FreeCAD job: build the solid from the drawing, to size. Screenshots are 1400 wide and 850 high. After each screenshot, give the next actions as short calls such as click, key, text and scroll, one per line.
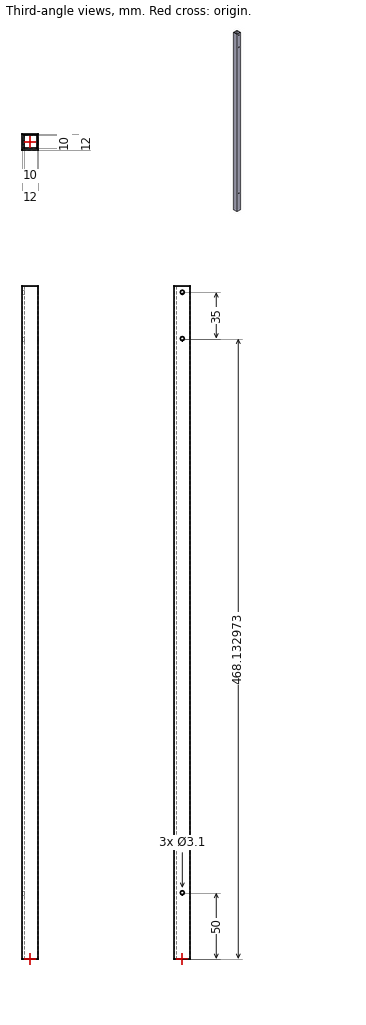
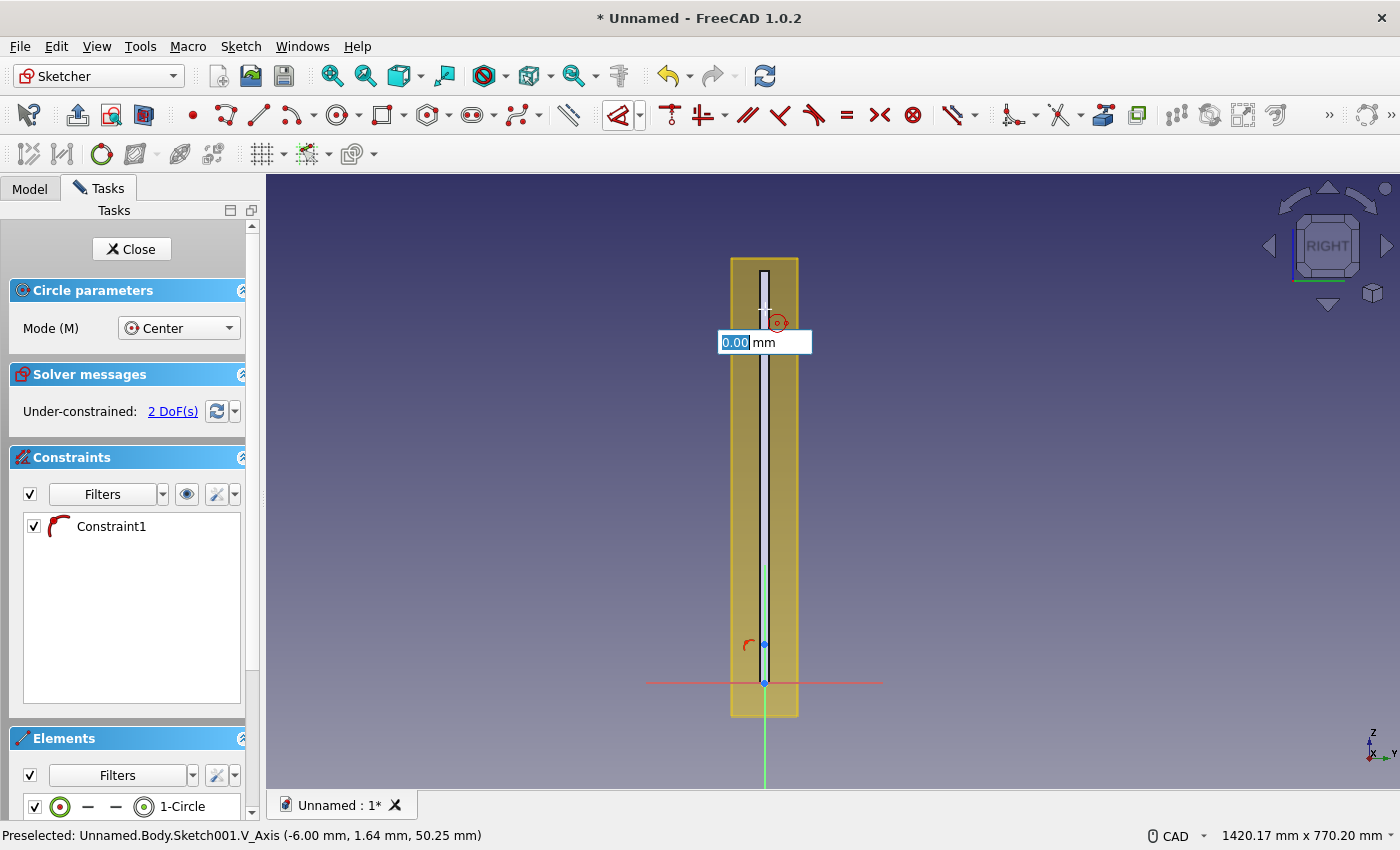
scroll(766, 309, up, 14)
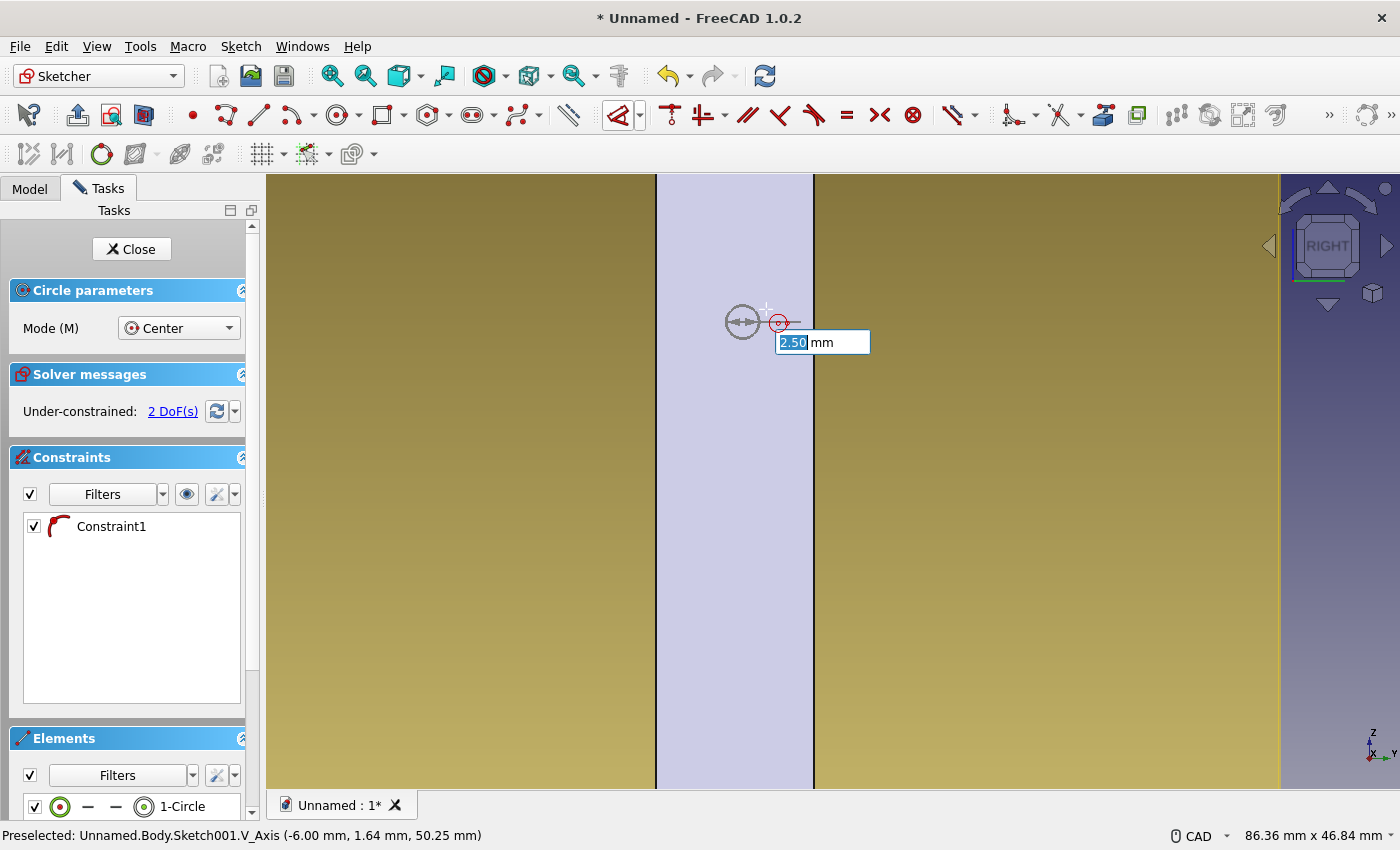
click(754, 306)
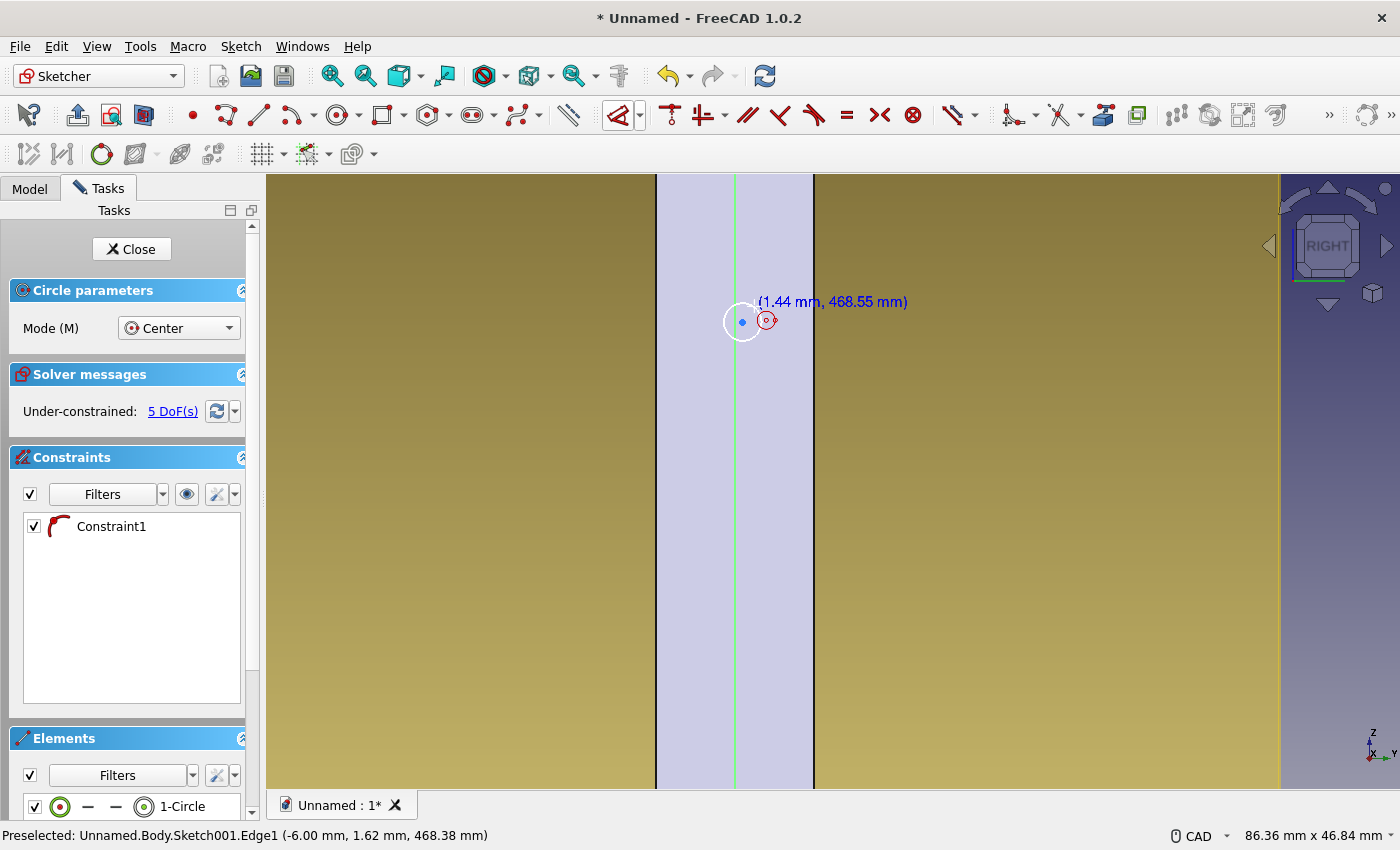
scroll(766, 309, down, 14)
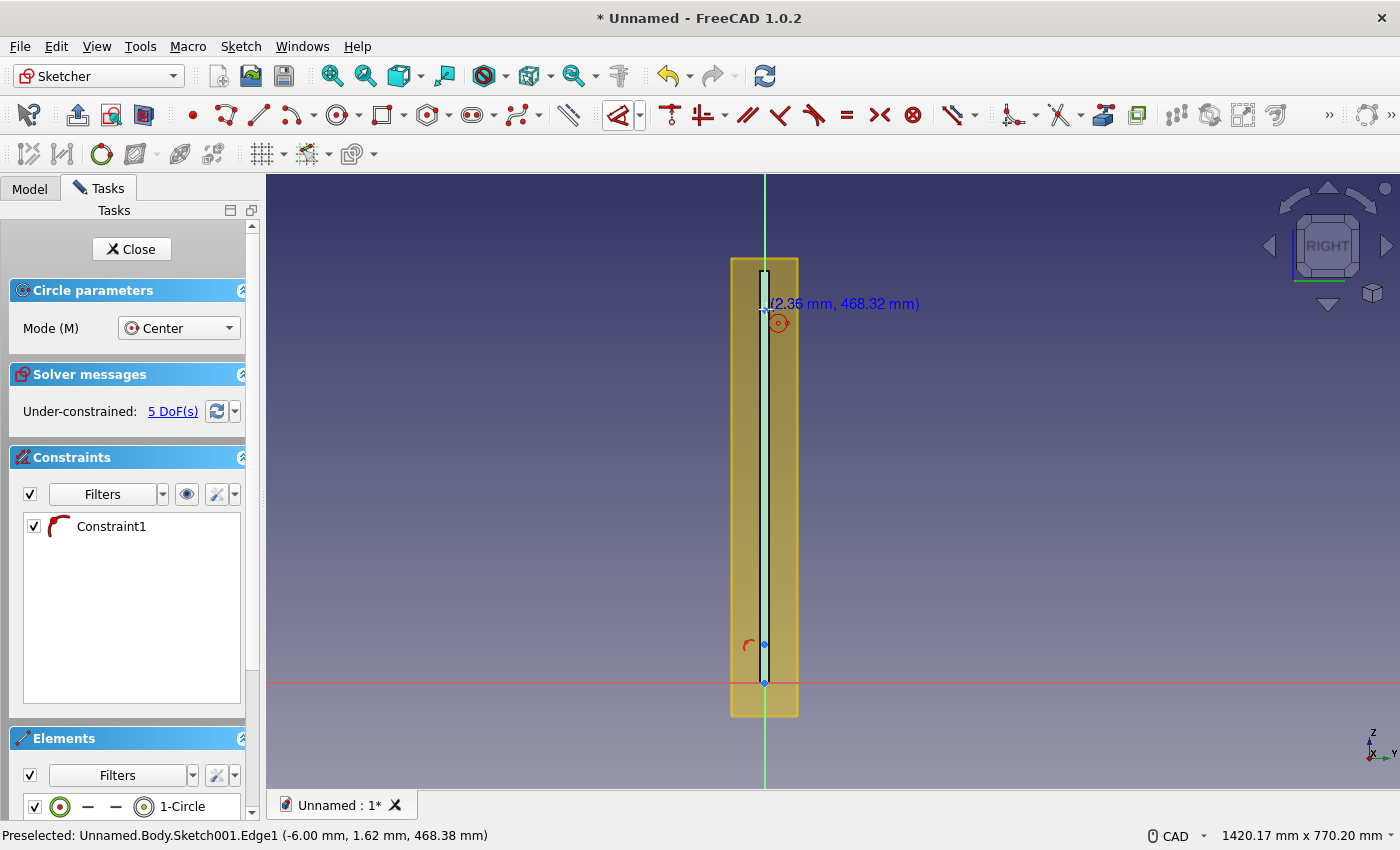
scroll(765, 281, up, 15)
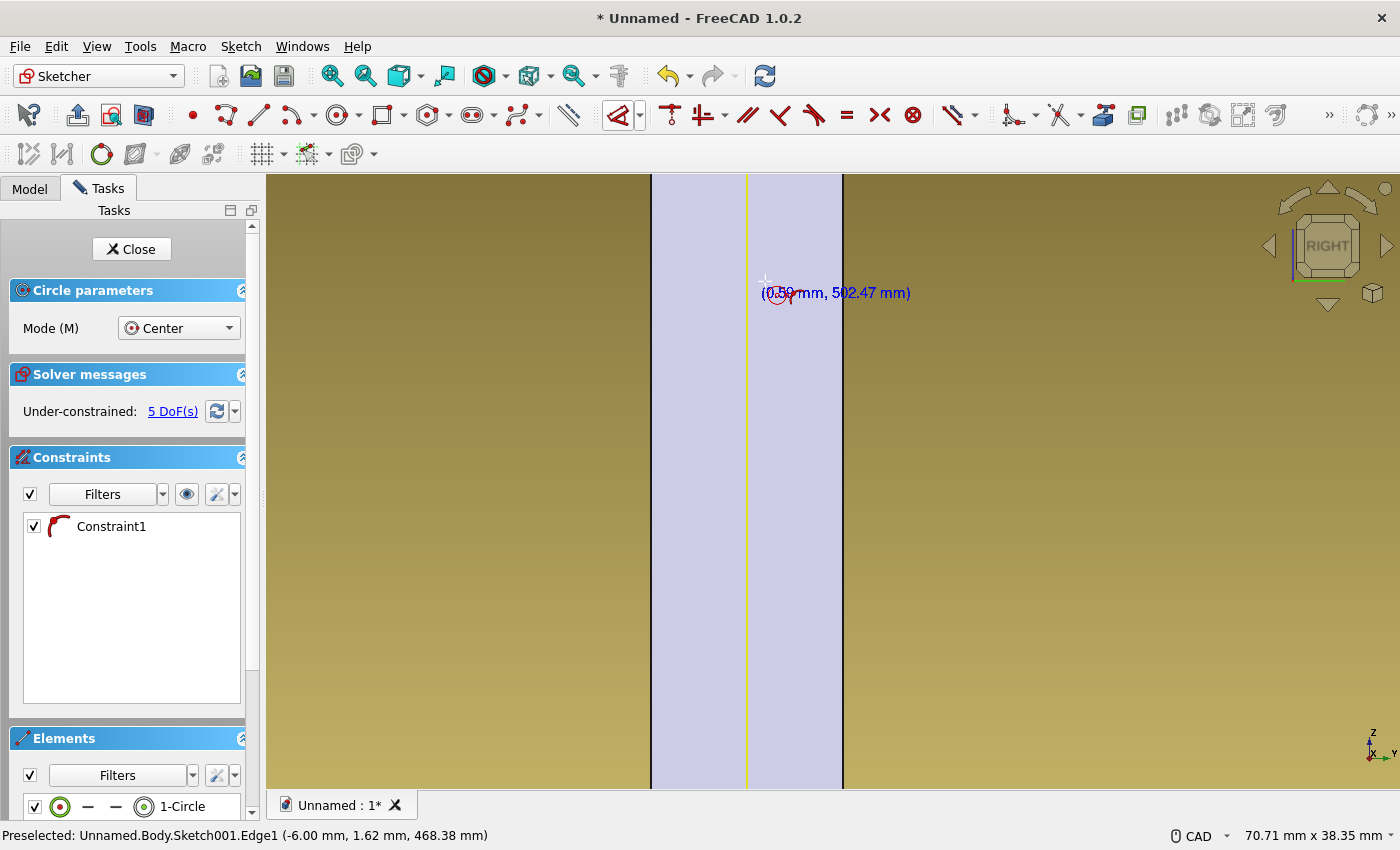
scroll(765, 281, down, 15)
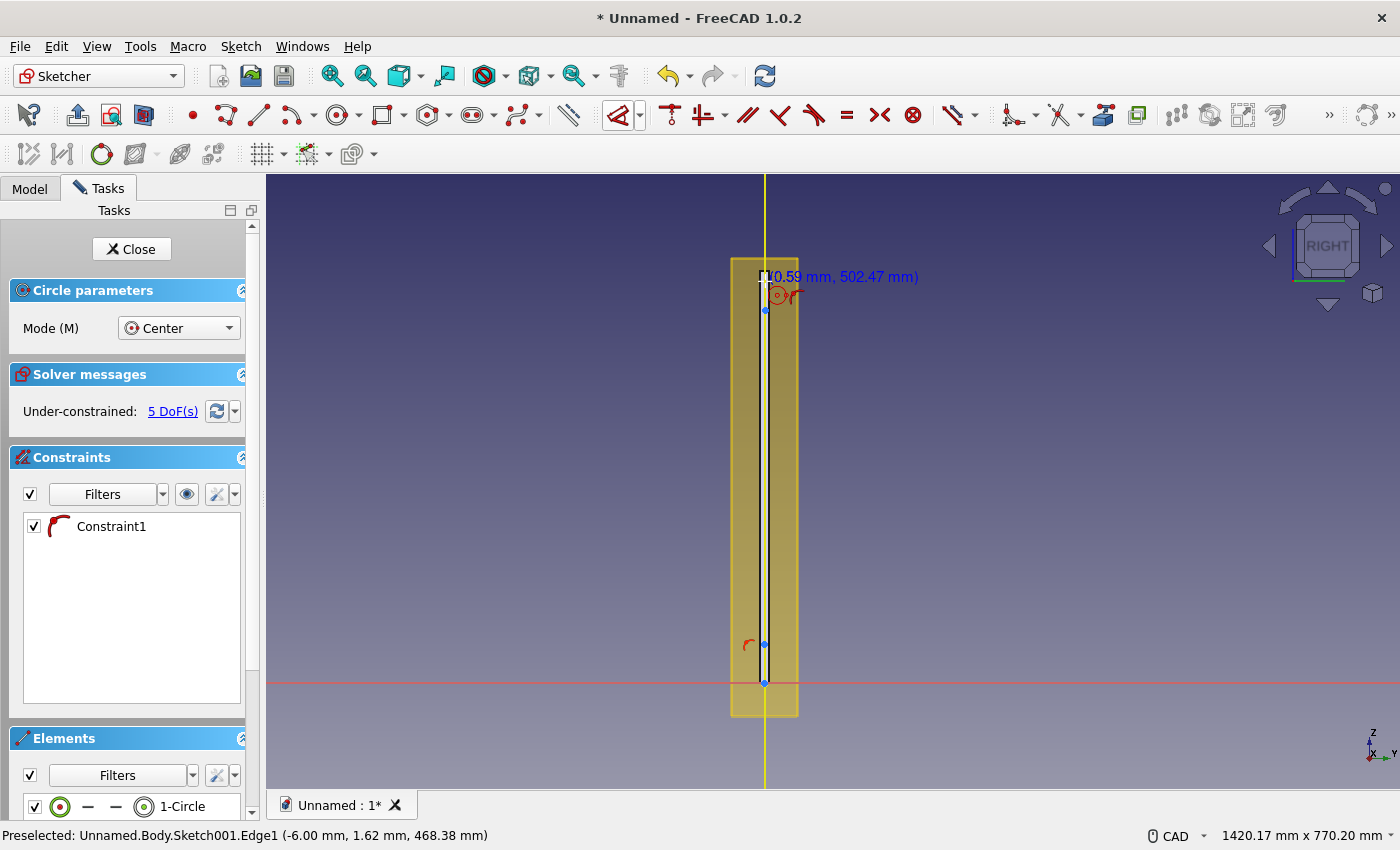
click(765, 281)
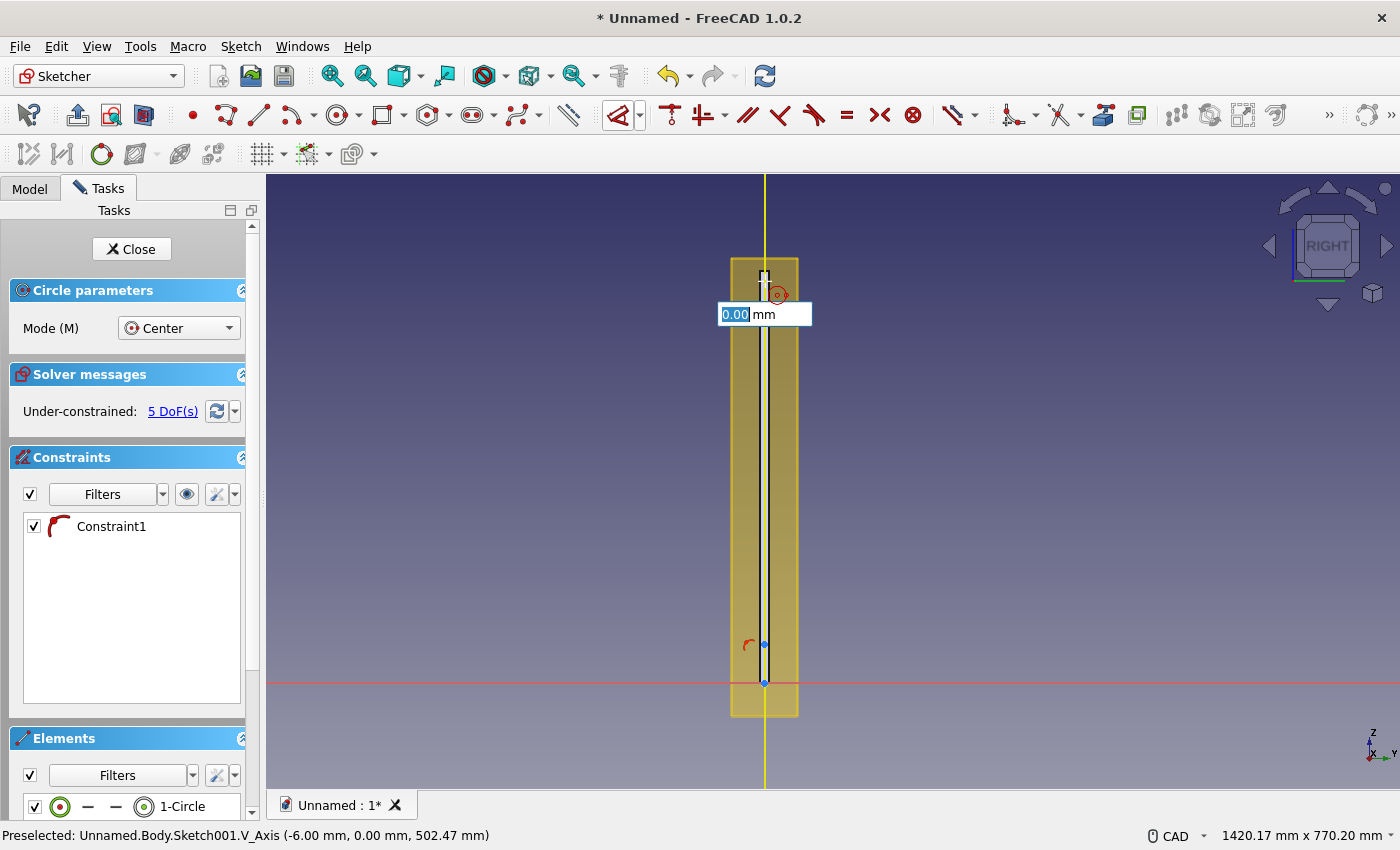
scroll(766, 281, up, 14)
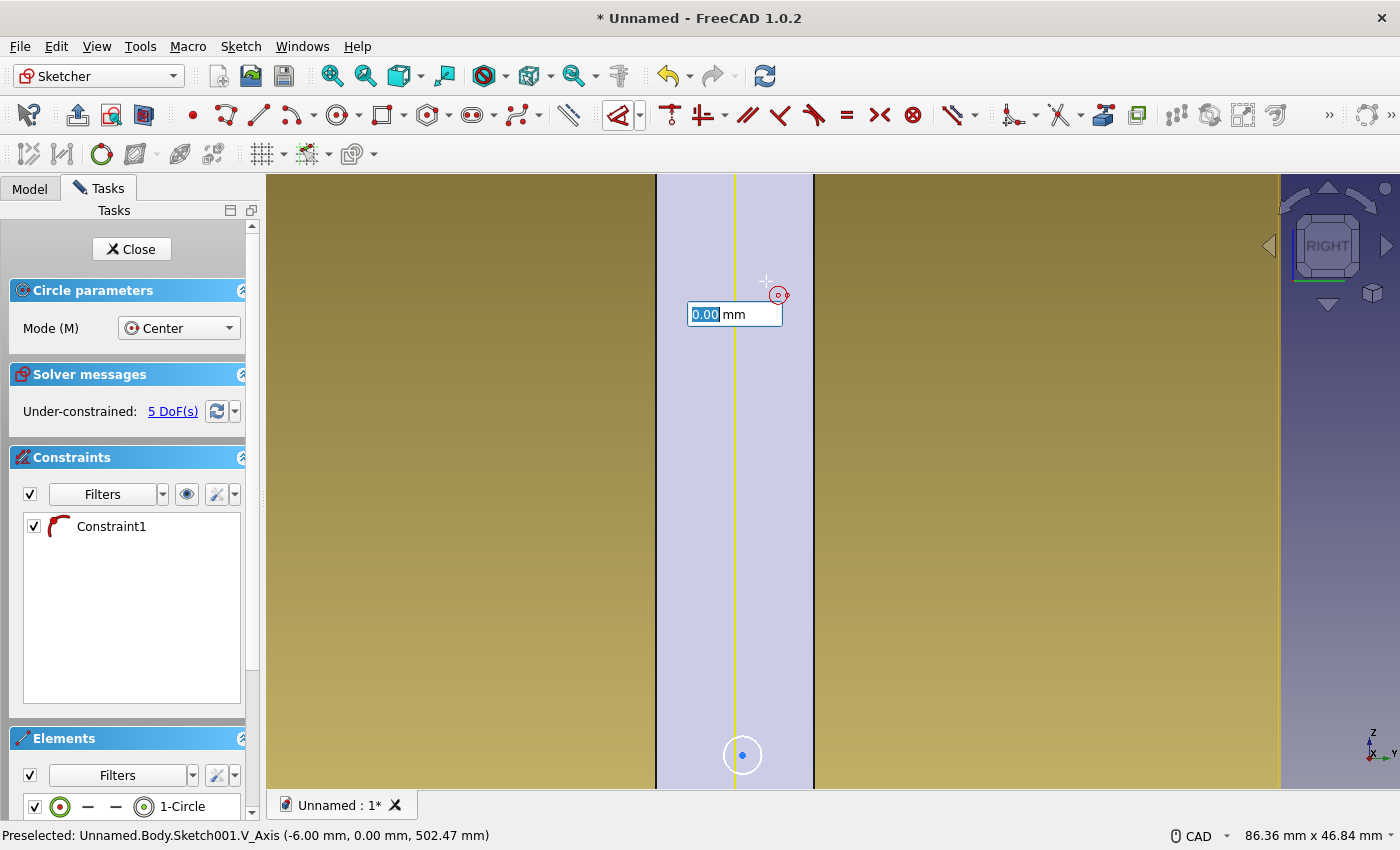
click(754, 279)
key(Escape)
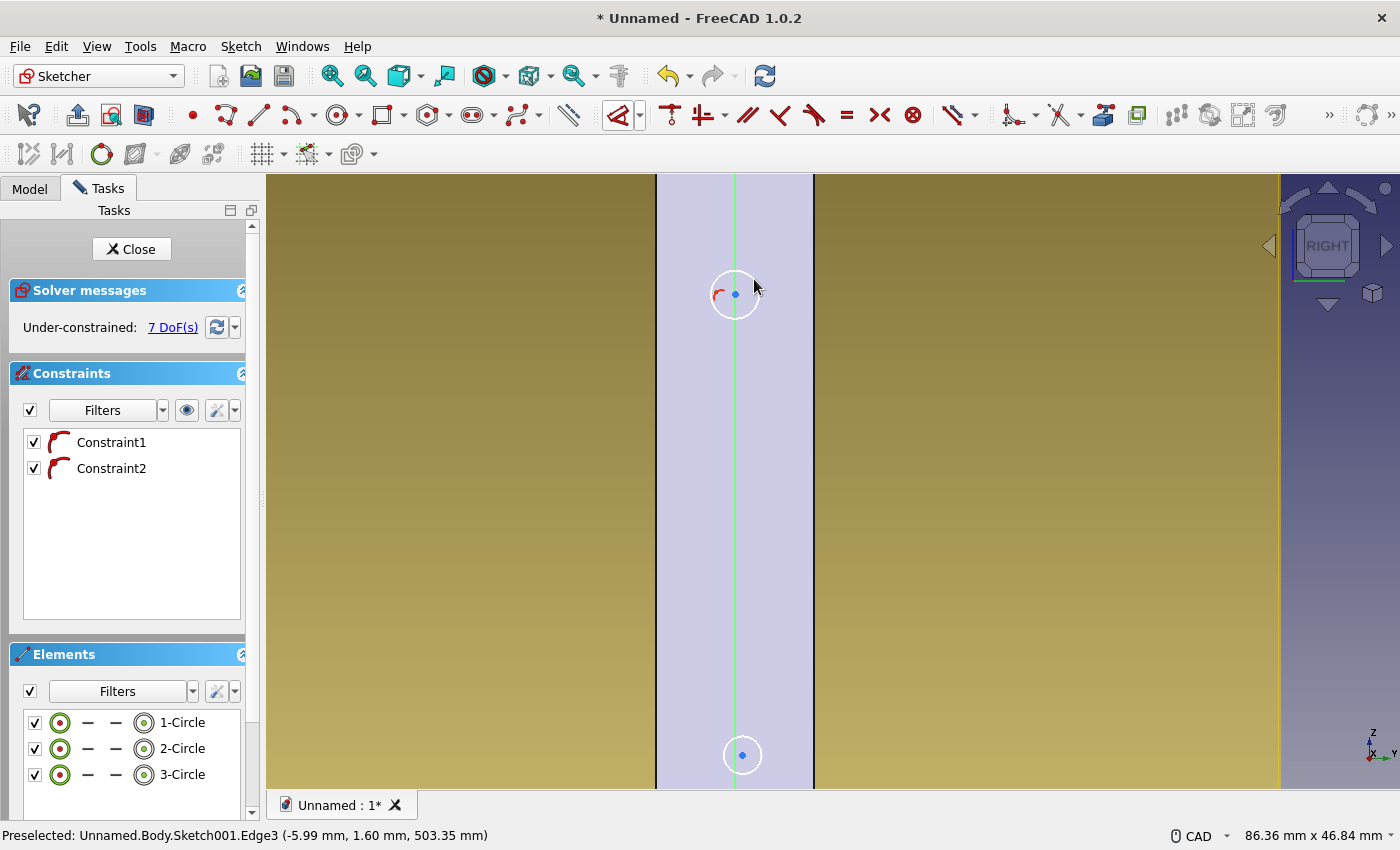
scroll(766, 281, down, 14)